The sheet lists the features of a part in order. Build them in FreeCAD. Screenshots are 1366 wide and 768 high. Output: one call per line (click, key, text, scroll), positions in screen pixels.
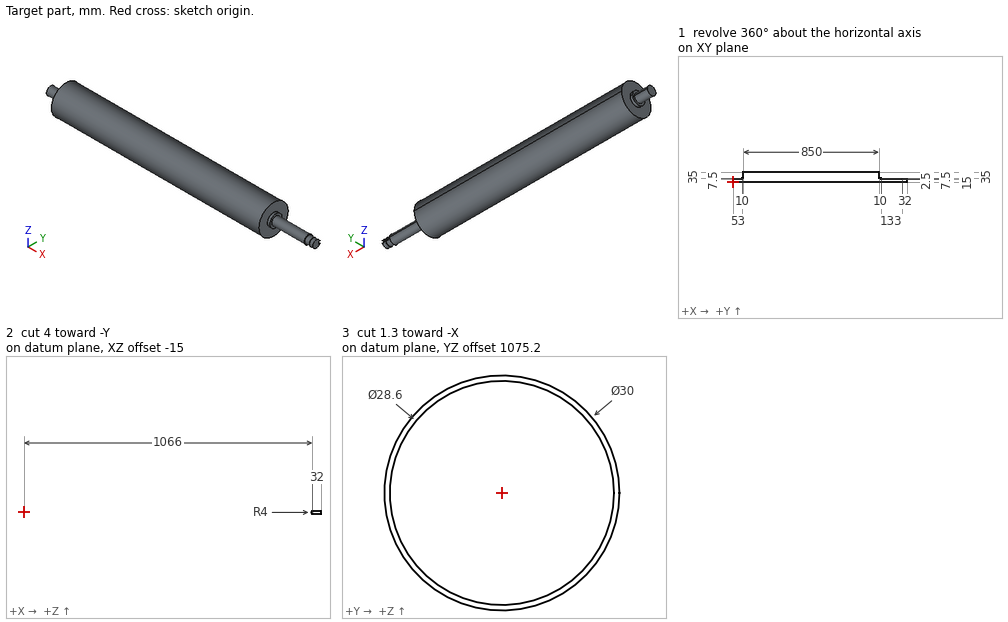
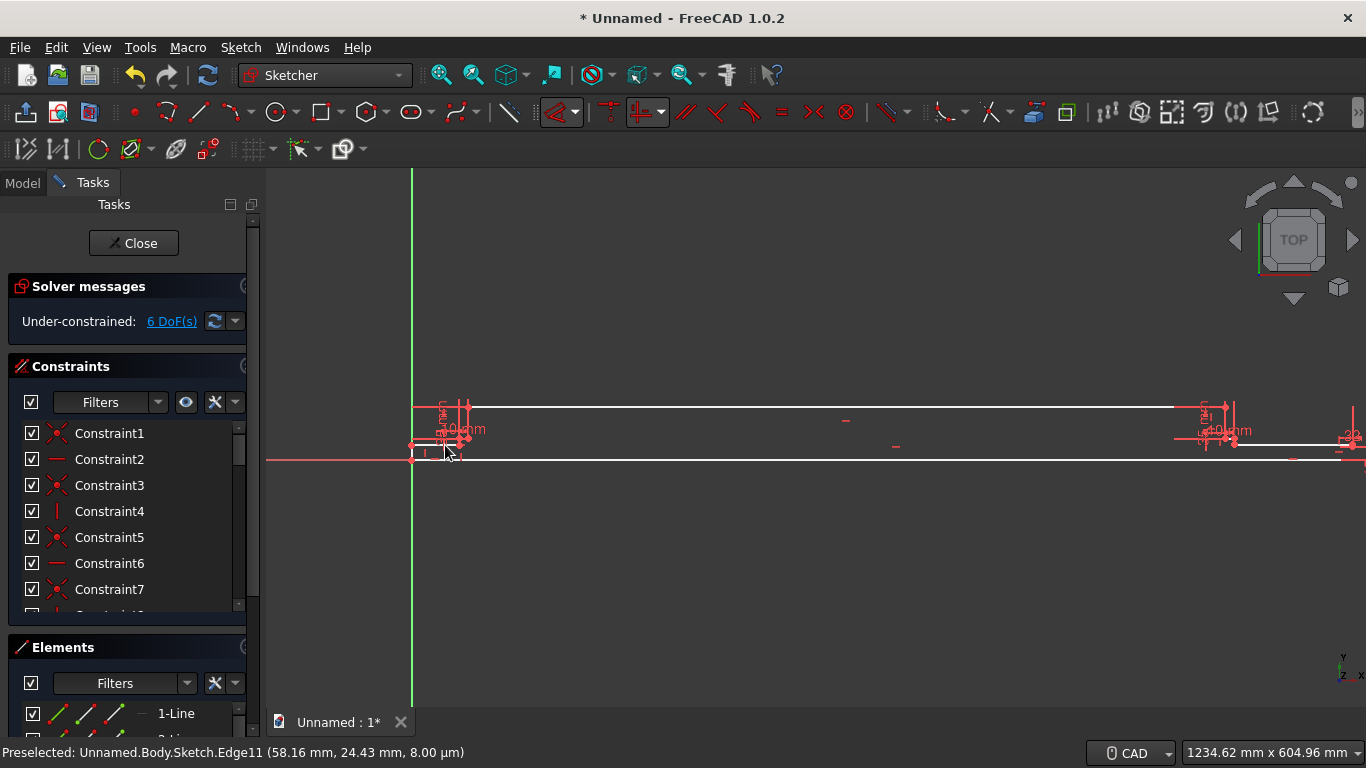
click(445, 445)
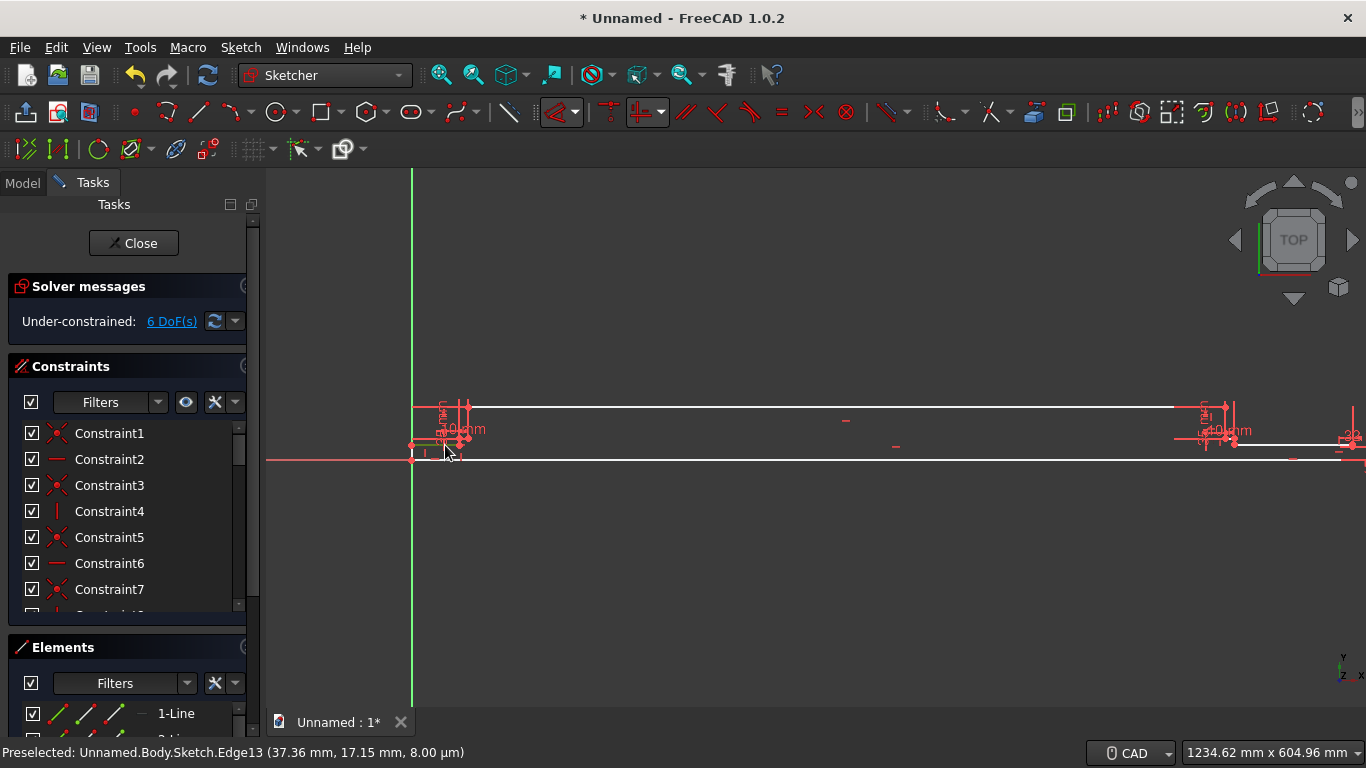
click(578, 112)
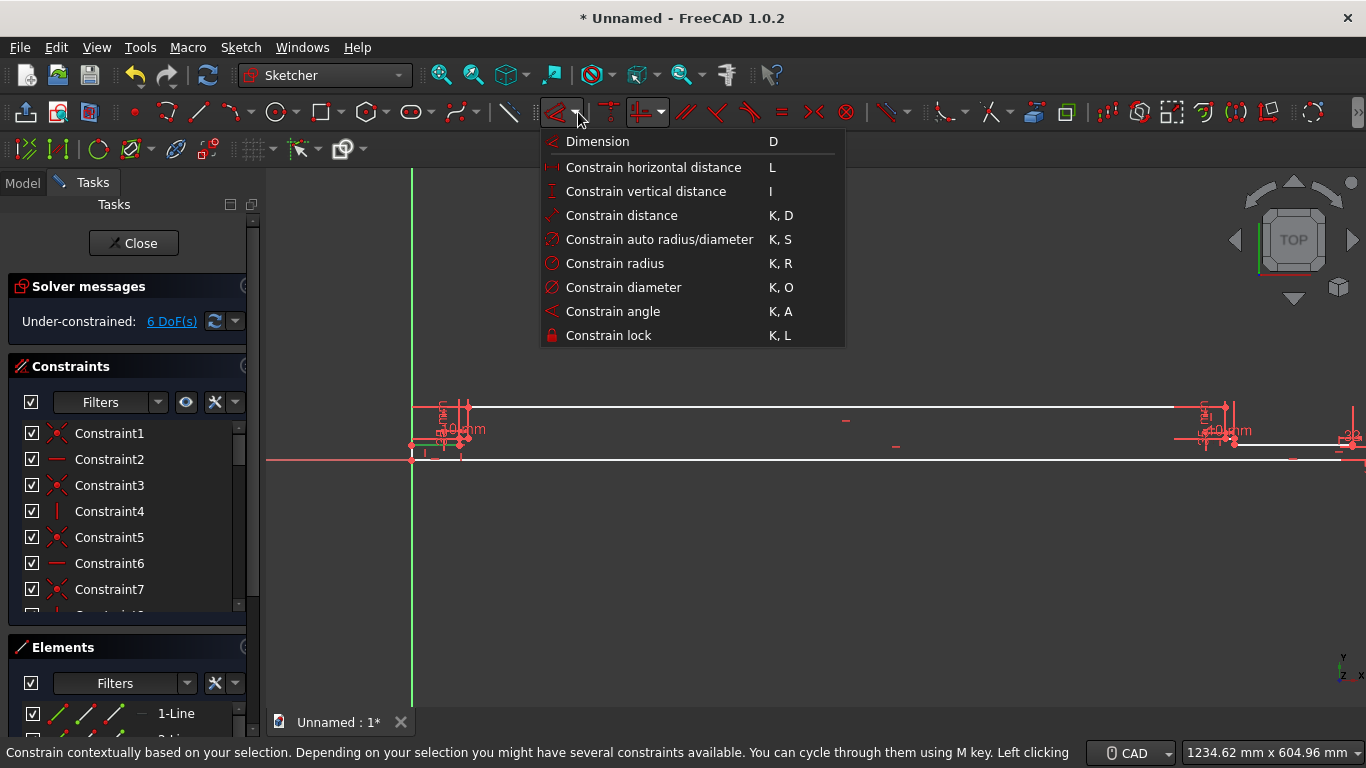
click(693, 167)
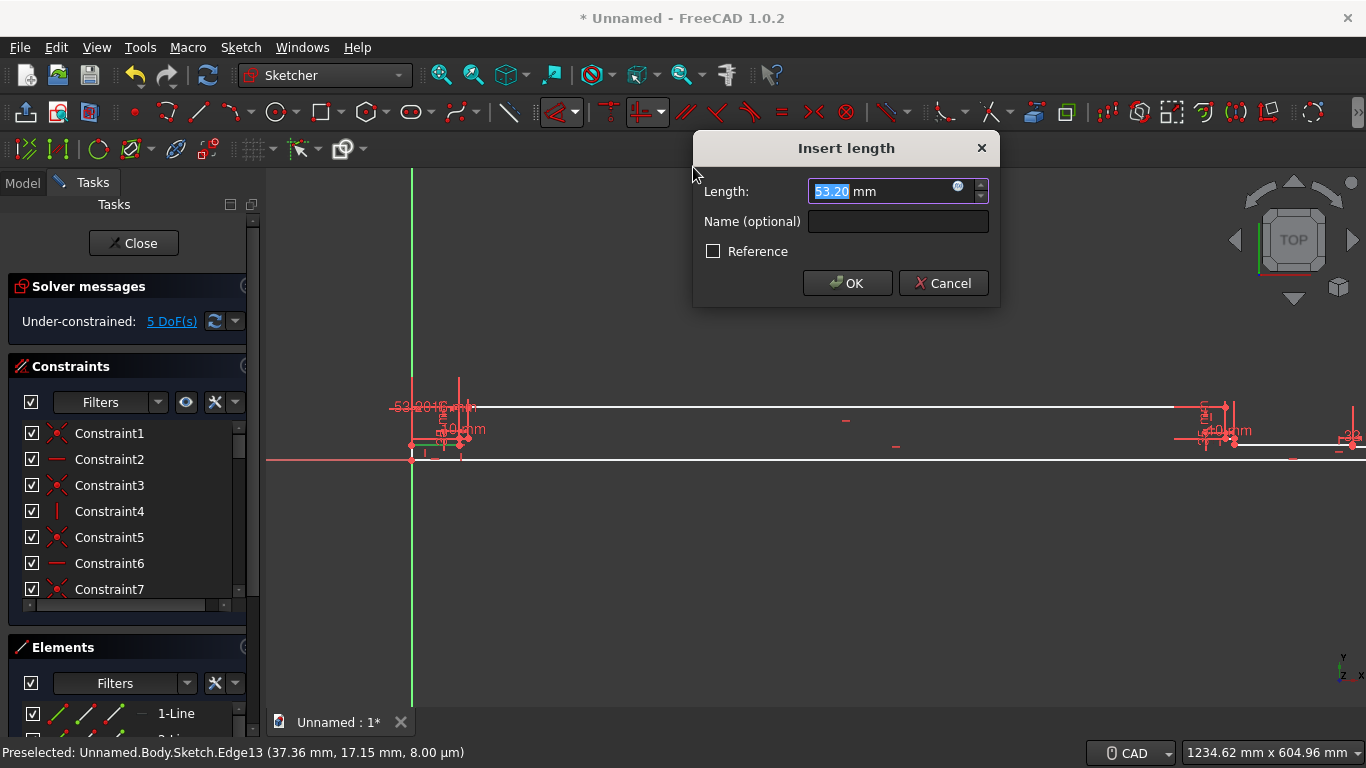
text(53)
key(Return)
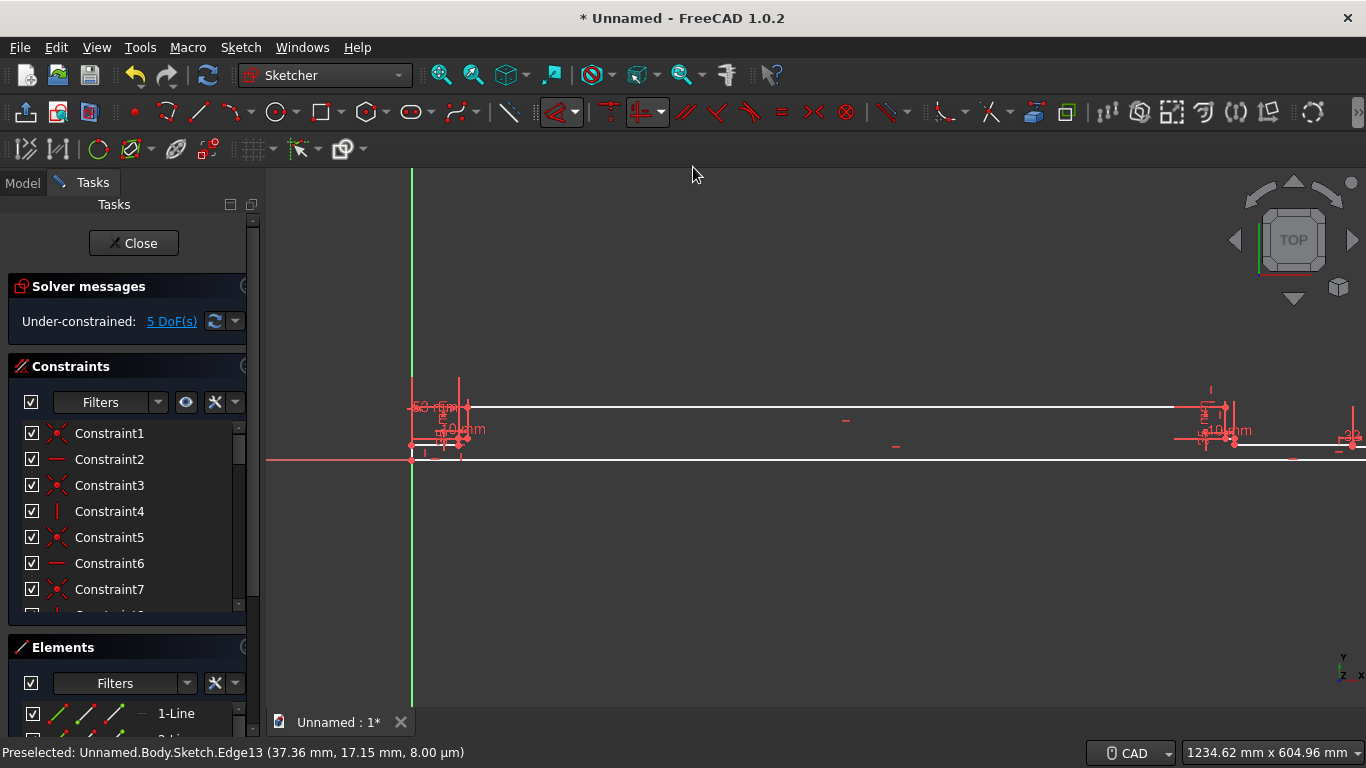
scroll(445, 446, down, 2)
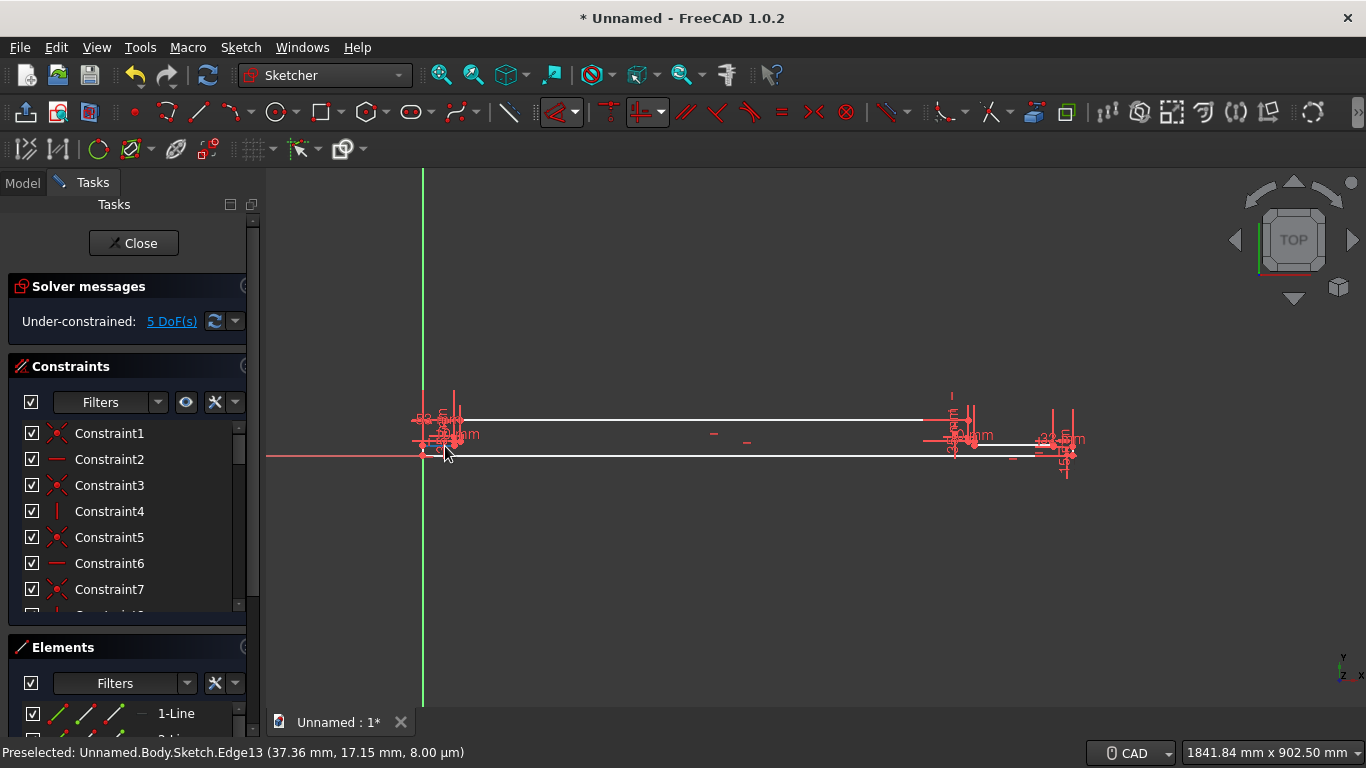
scroll(1053, 446, up, 17)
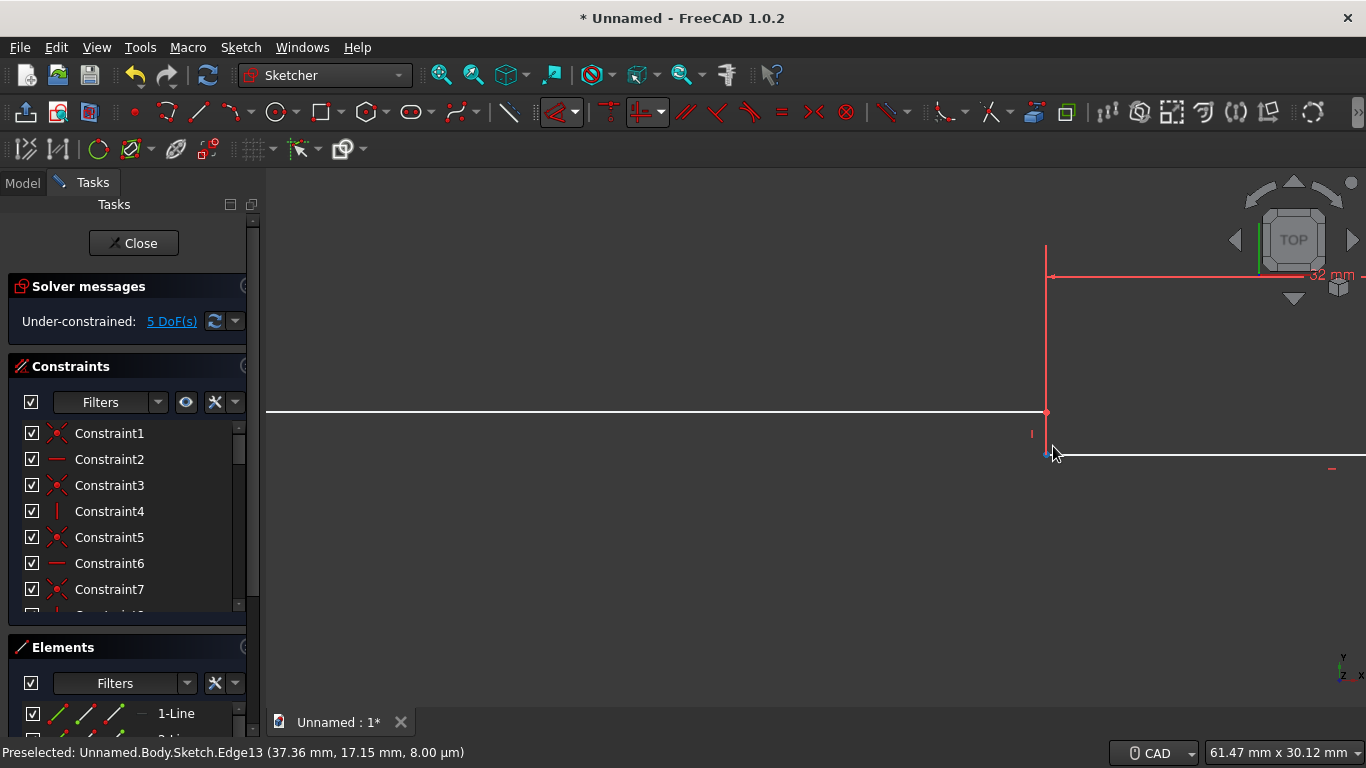
click(1046, 433)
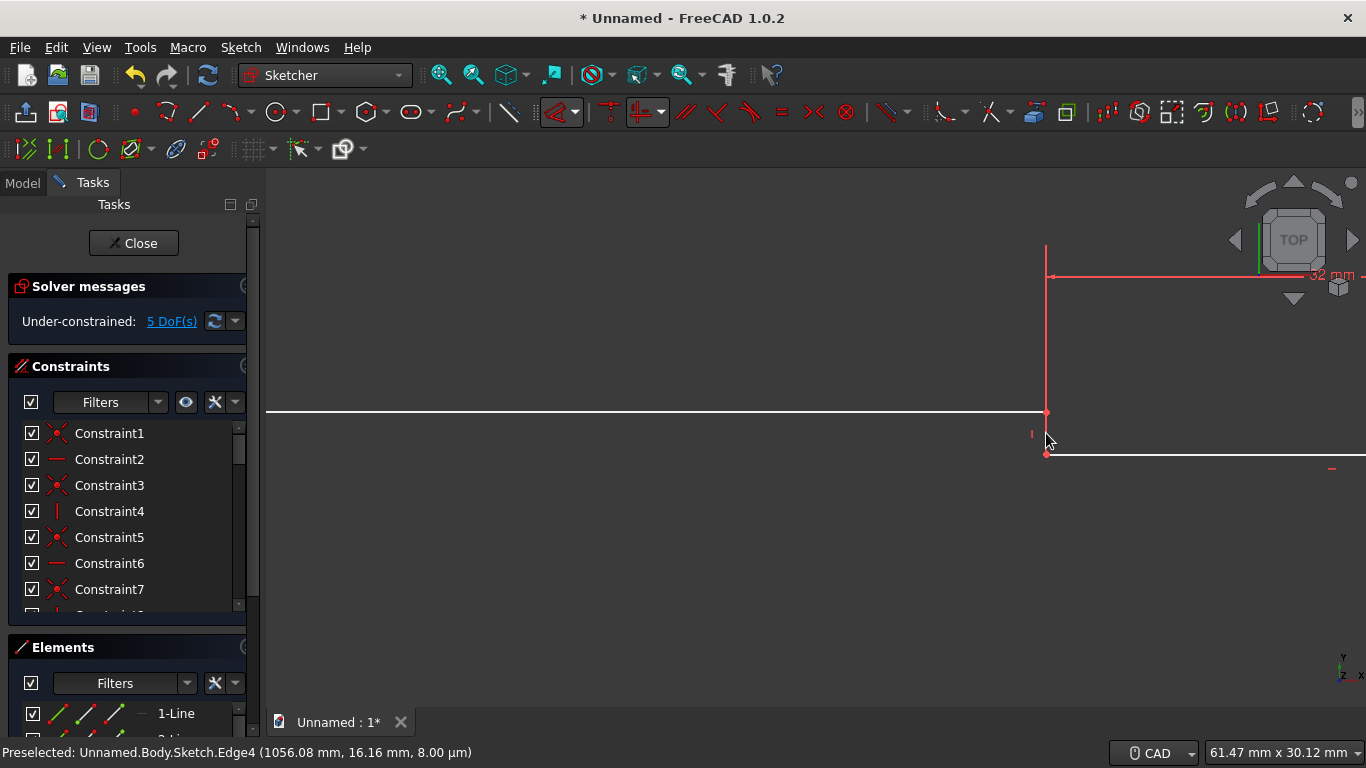
click(578, 112)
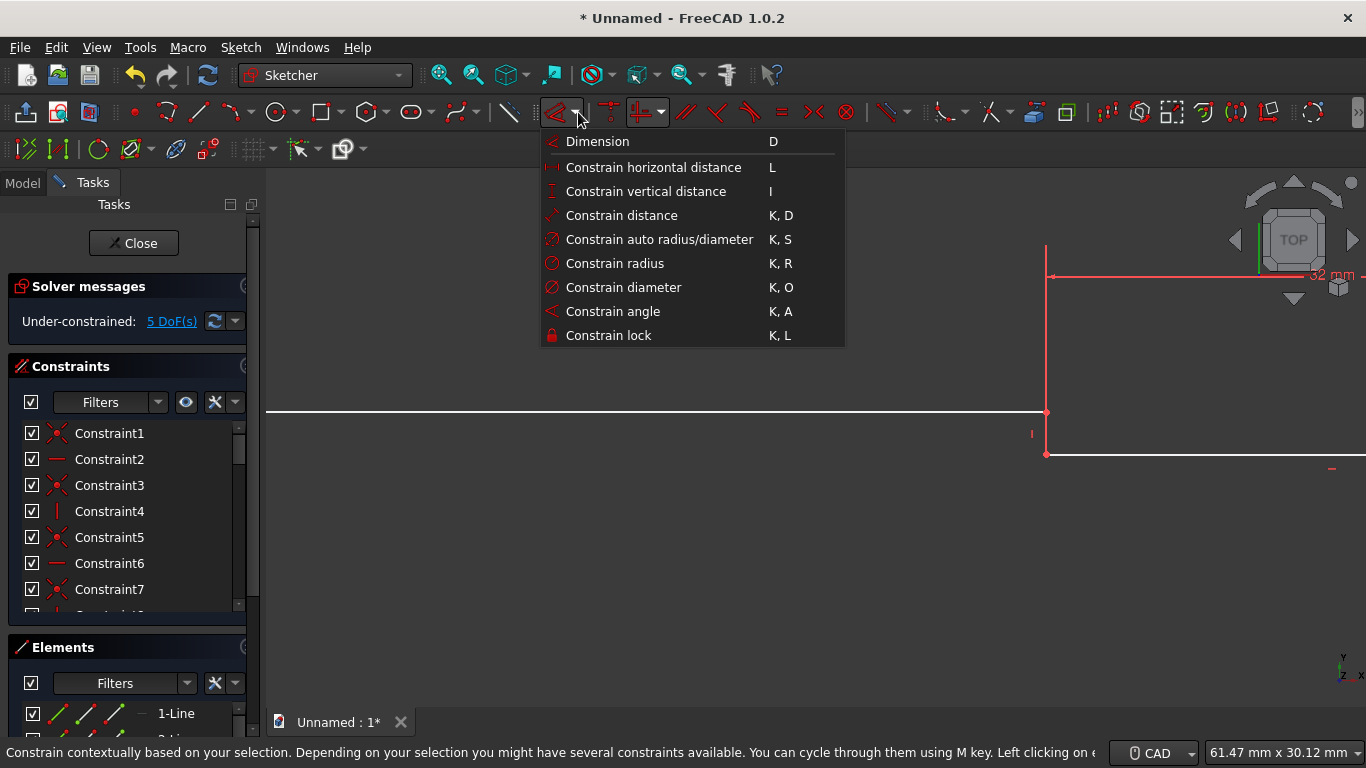
click(693, 191)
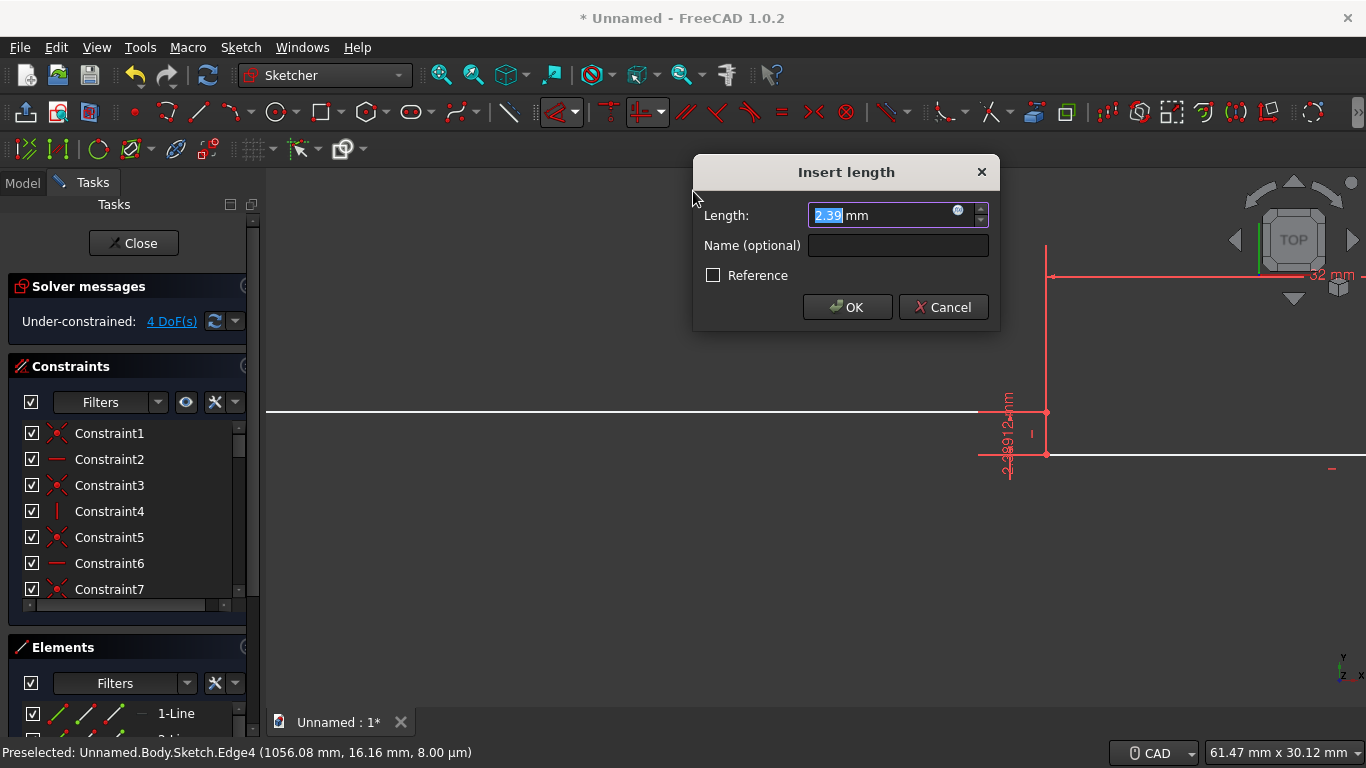
text(2.5)
key(Return)